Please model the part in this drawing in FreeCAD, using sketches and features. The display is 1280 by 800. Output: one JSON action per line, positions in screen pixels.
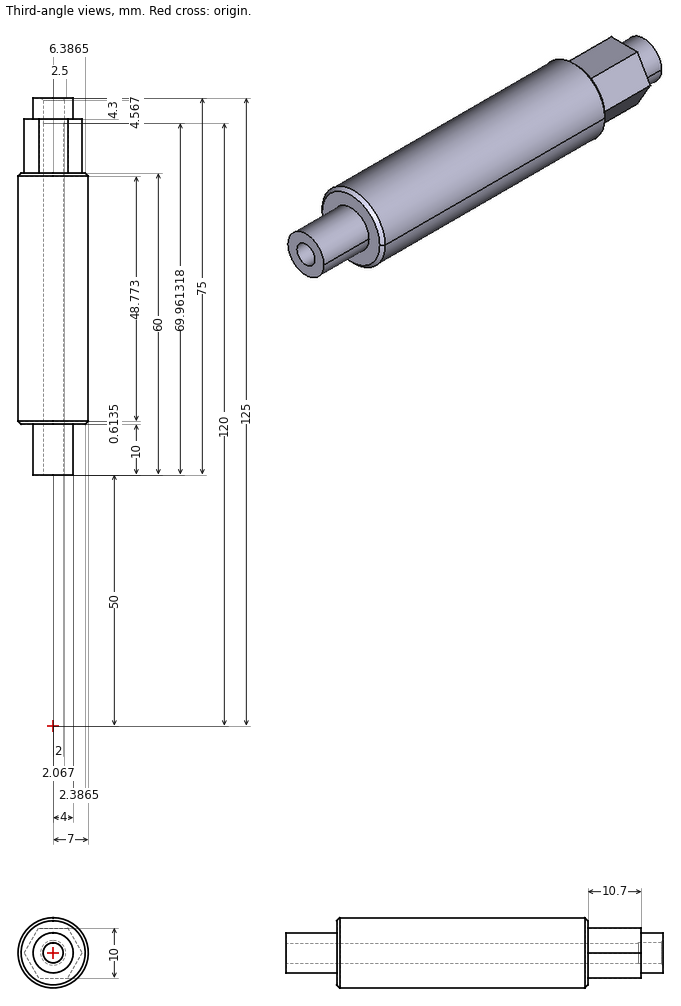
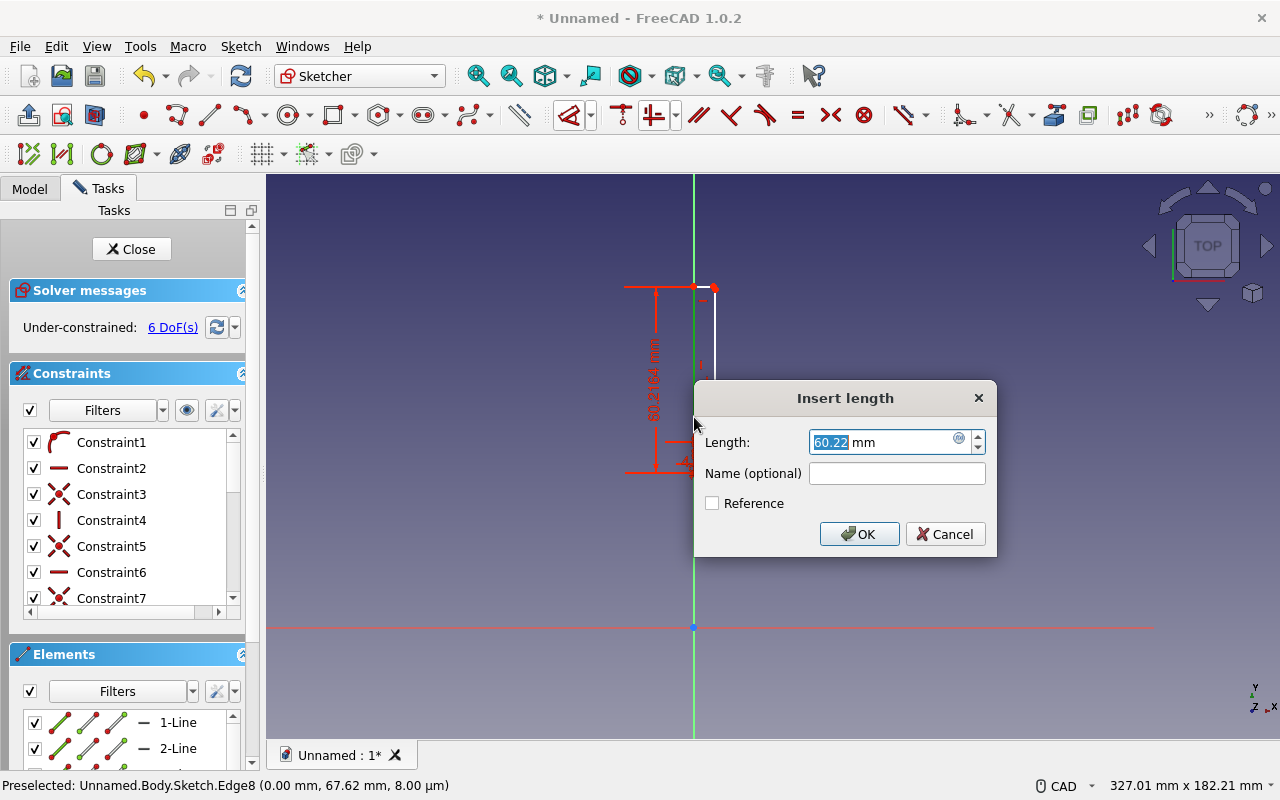
{"action": "type", "text": "60"}
{"action": "key", "text": "Return"}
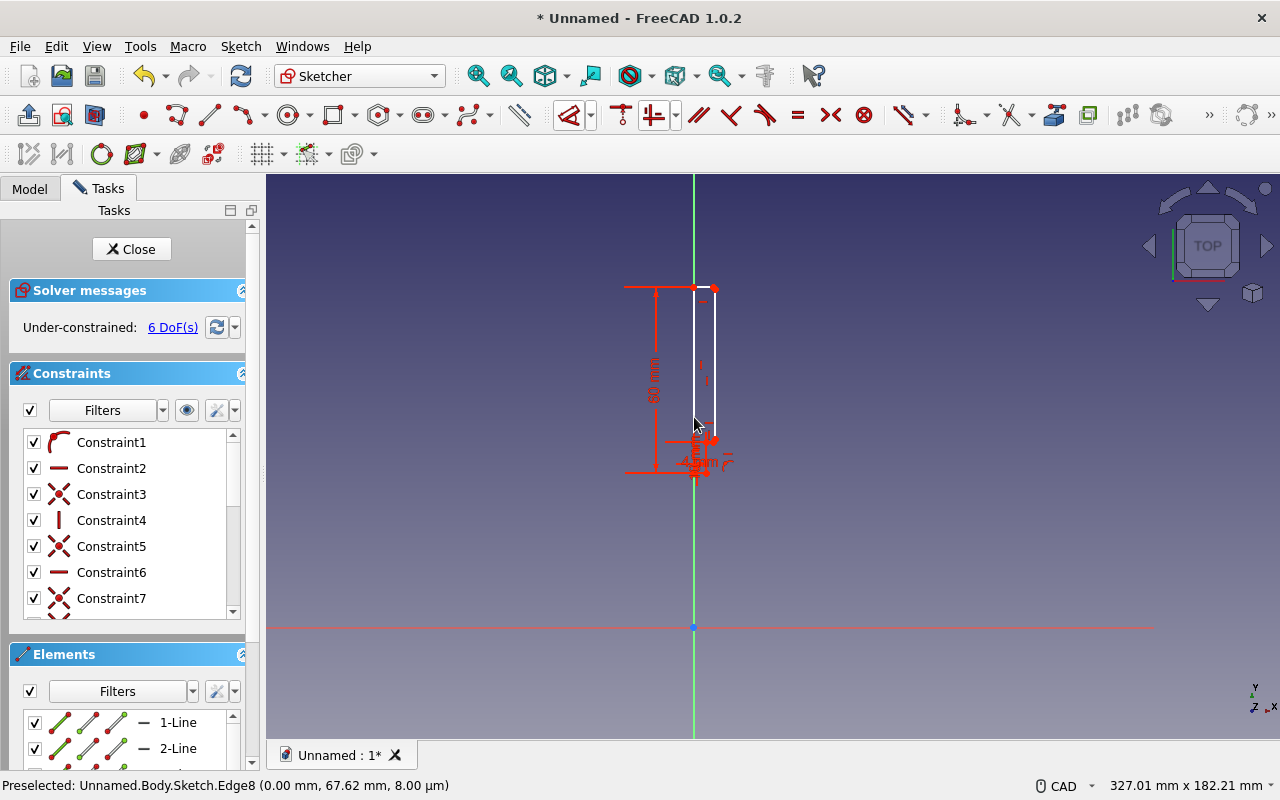
{"action": "scroll", "coordinate": [715, 440], "scroll_direction": "up", "scroll_amount": 7}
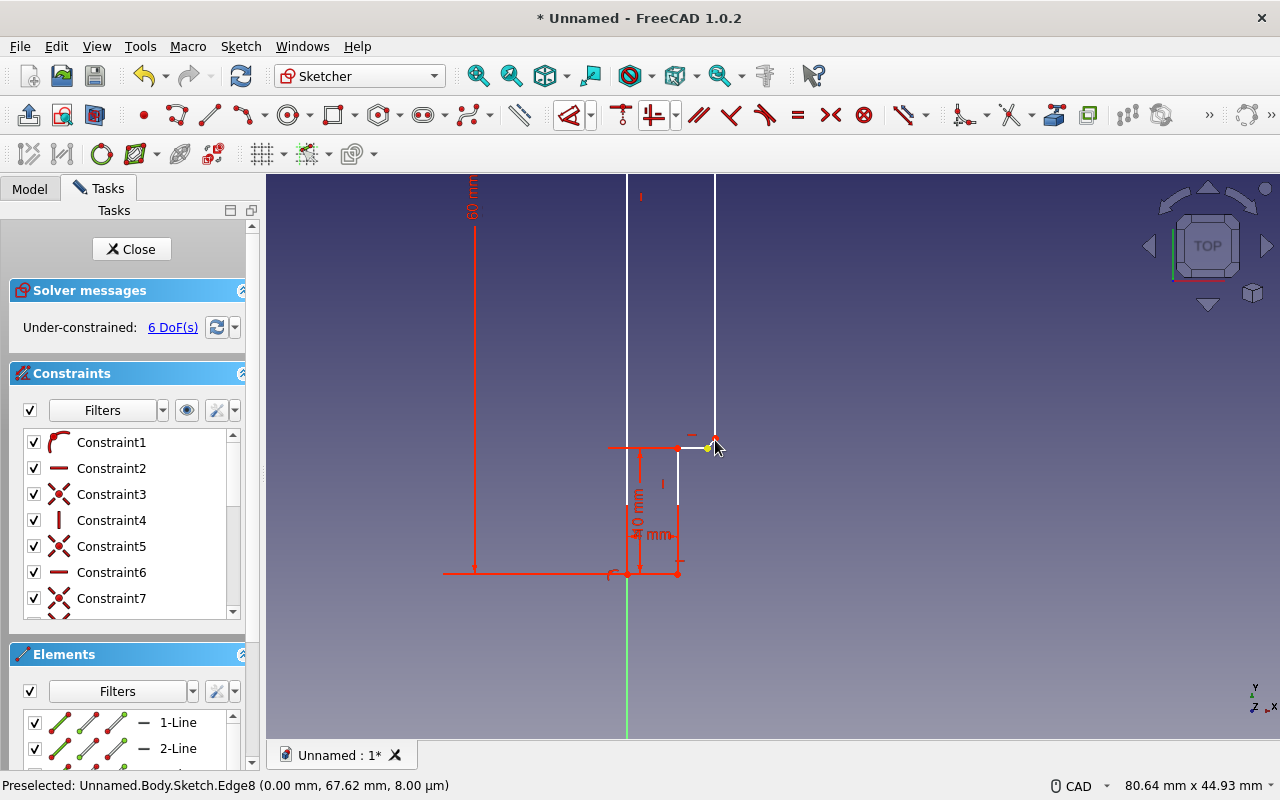
{"action": "left_click", "coordinate": [715, 438]}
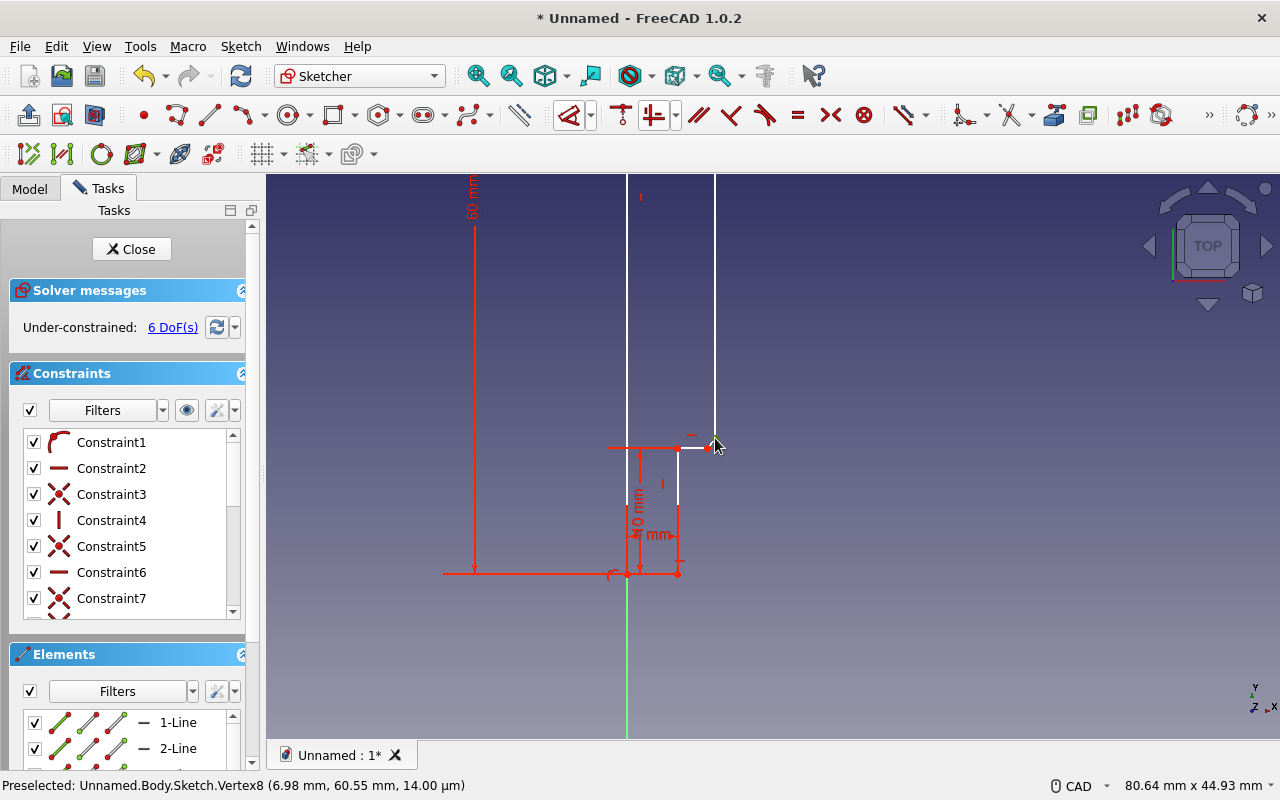
{"action": "left_click", "coordinate": [590, 116]}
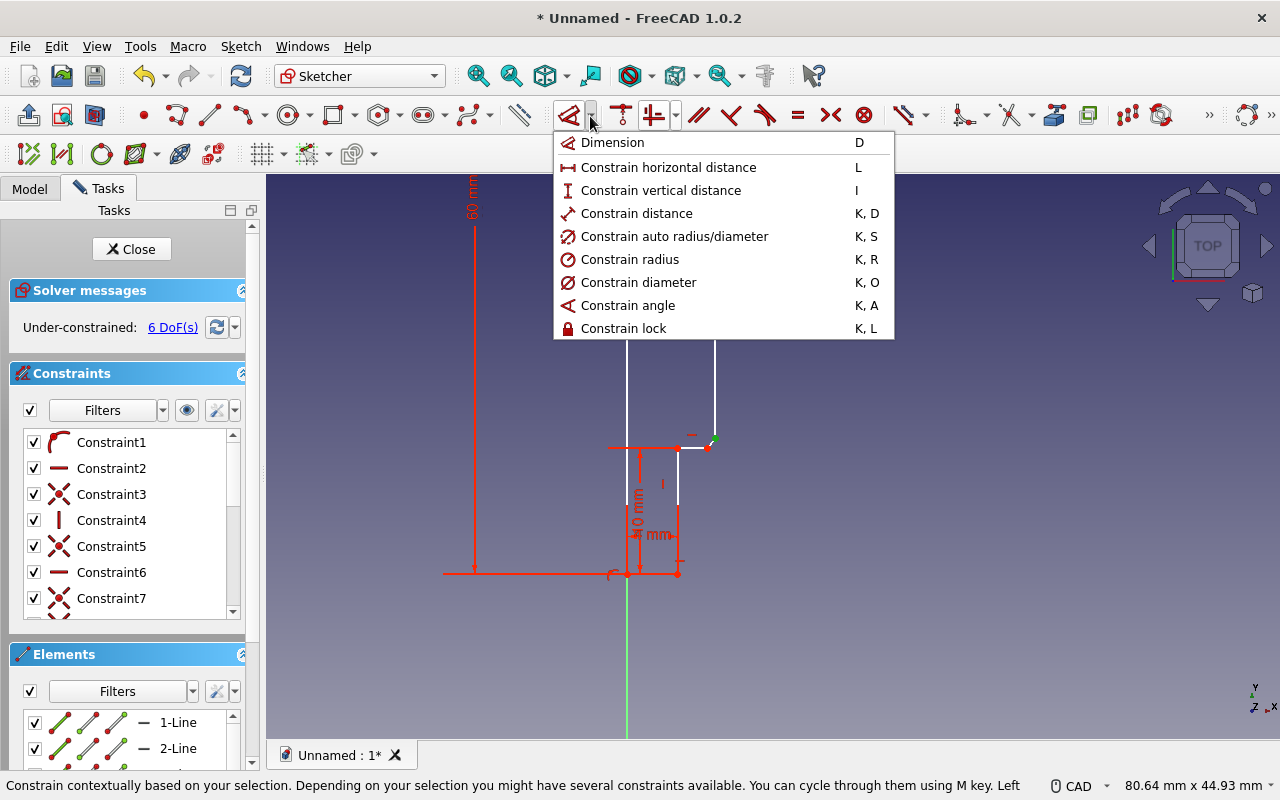
{"action": "left_click", "coordinate": [724, 168]}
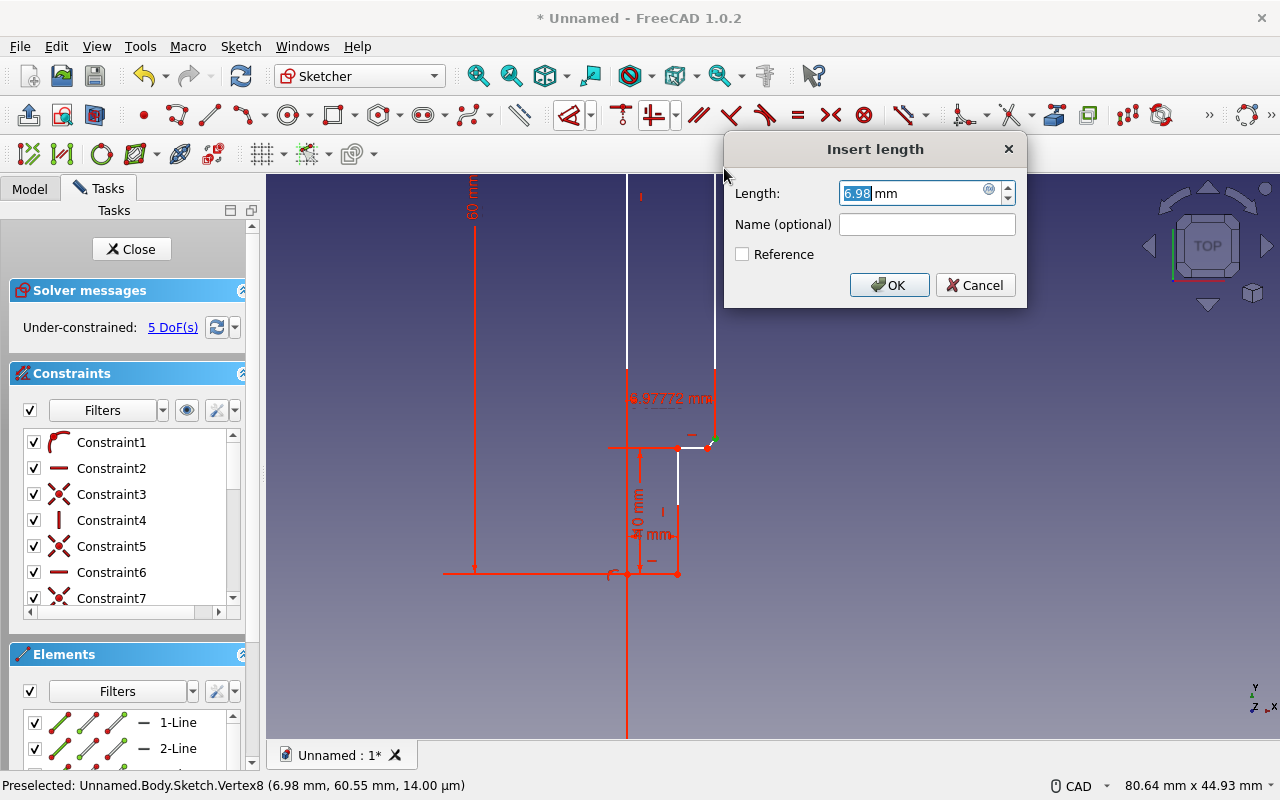
{"action": "type", "text": "7"}
{"action": "key", "text": "Return"}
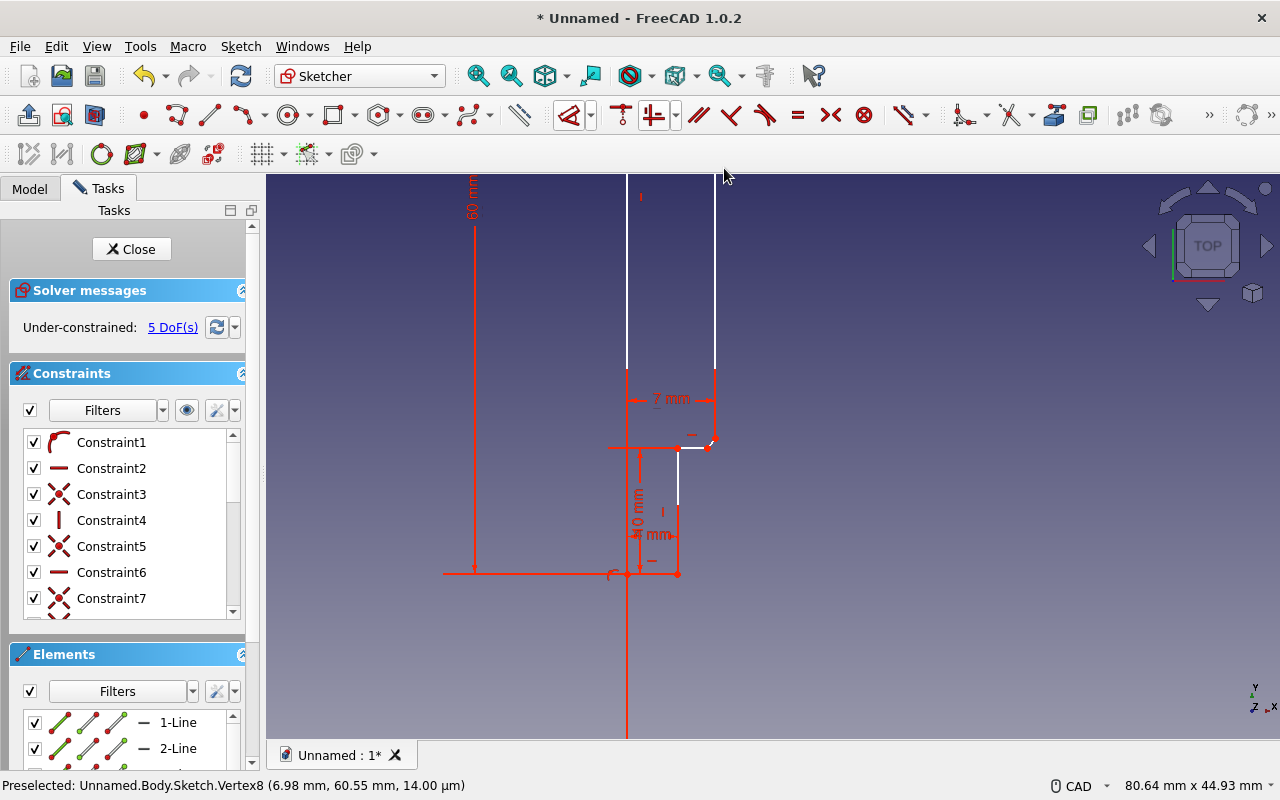
{"action": "scroll", "coordinate": [715, 440], "scroll_direction": "down", "scroll_amount": 7}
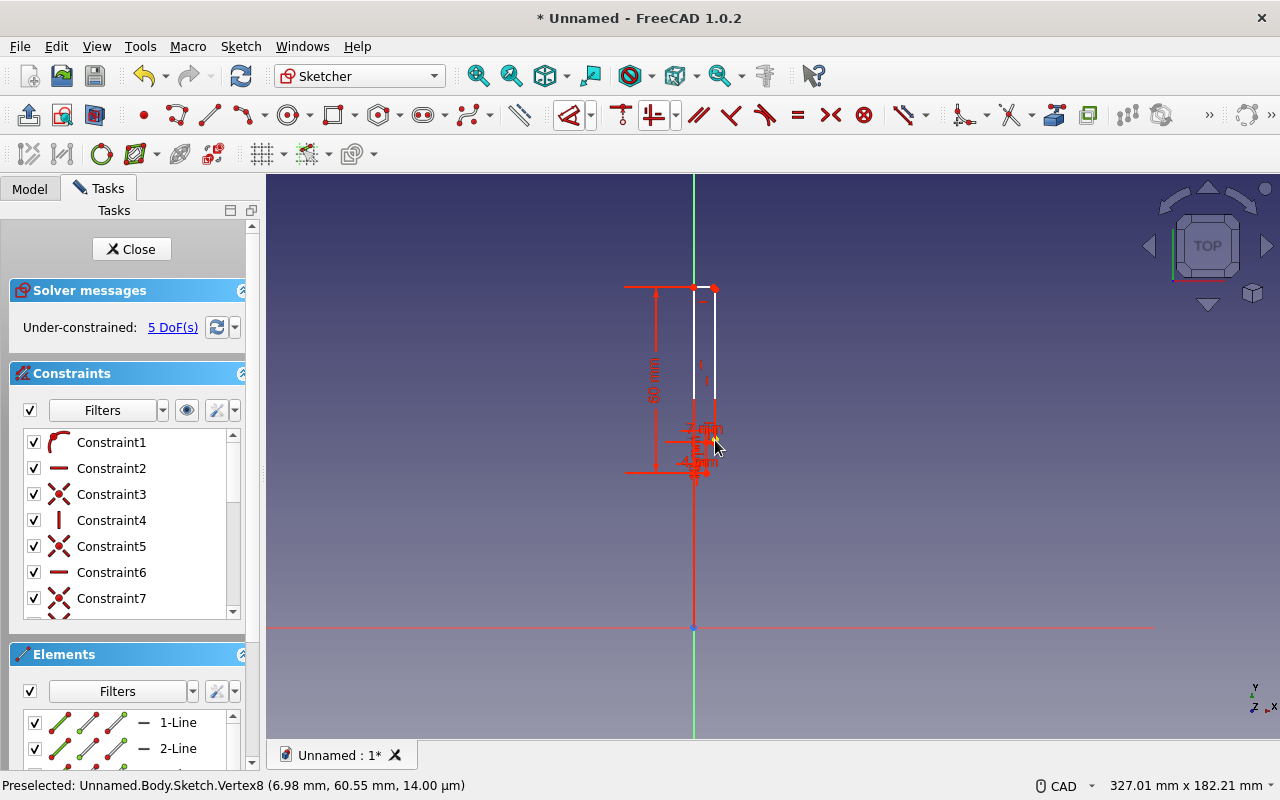
{"action": "left_click", "coordinate": [694, 473]}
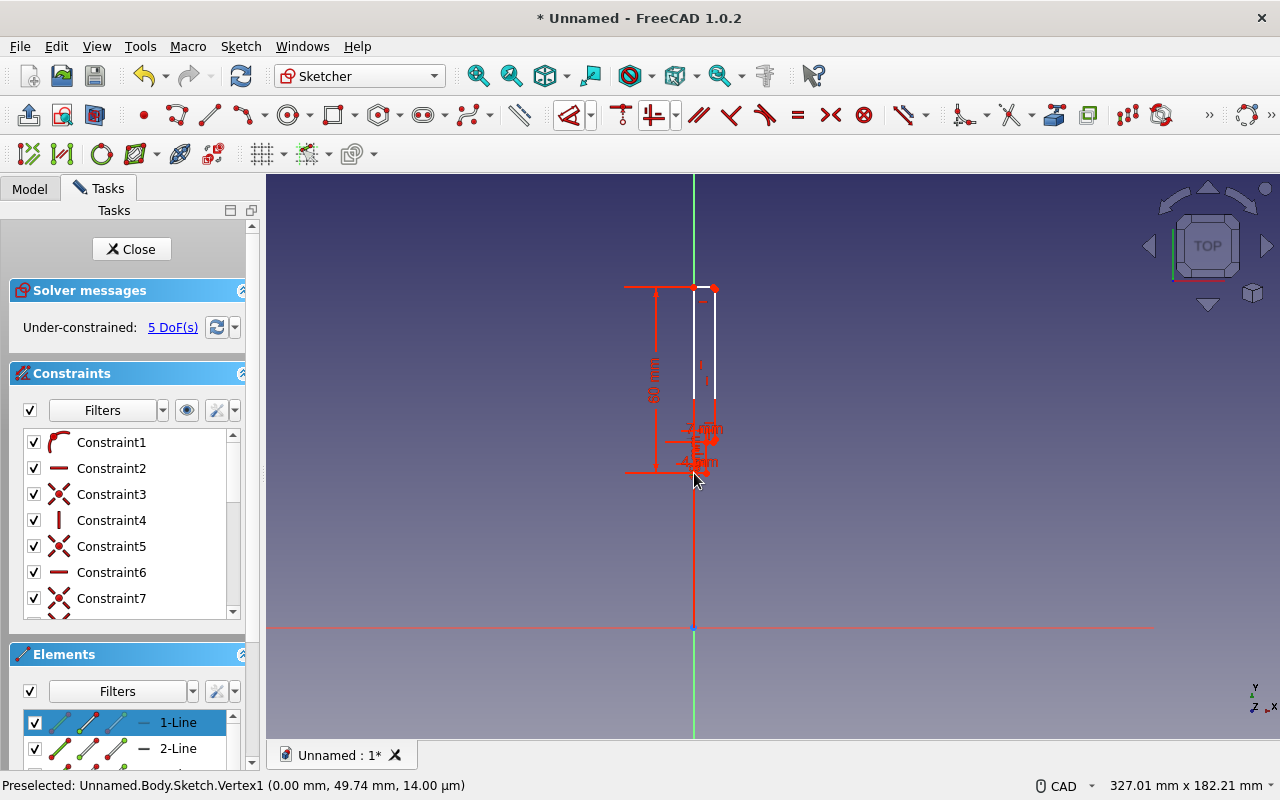
{"action": "key", "text": "i"}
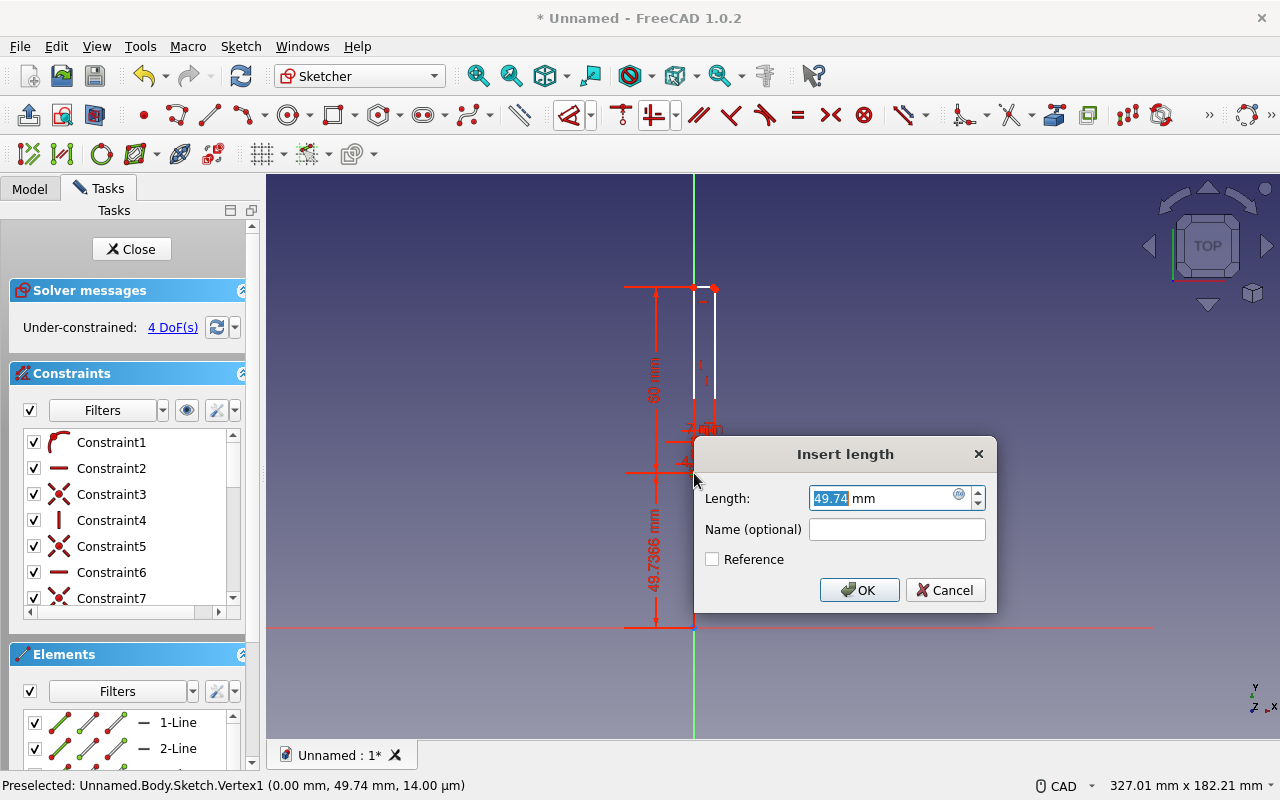
{"action": "type", "text": "50"}
{"action": "key", "text": "Return"}